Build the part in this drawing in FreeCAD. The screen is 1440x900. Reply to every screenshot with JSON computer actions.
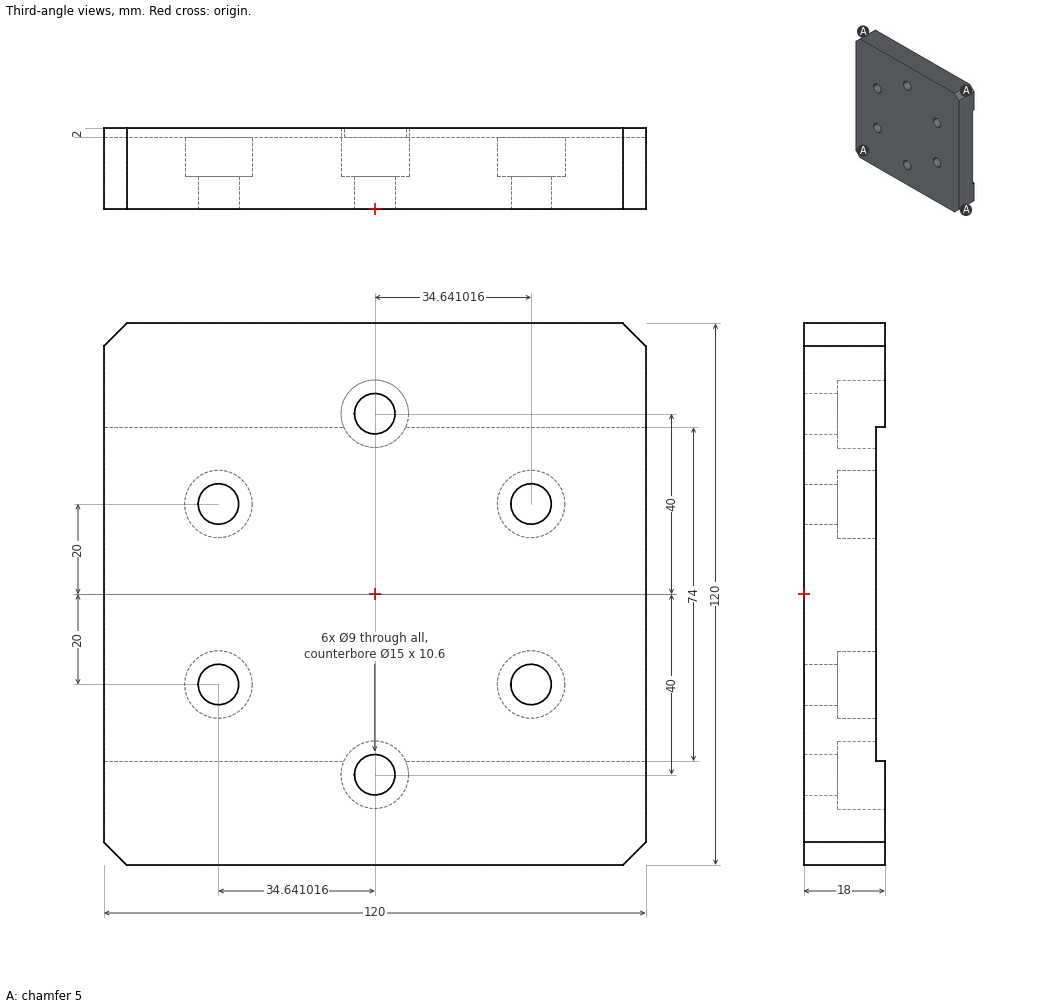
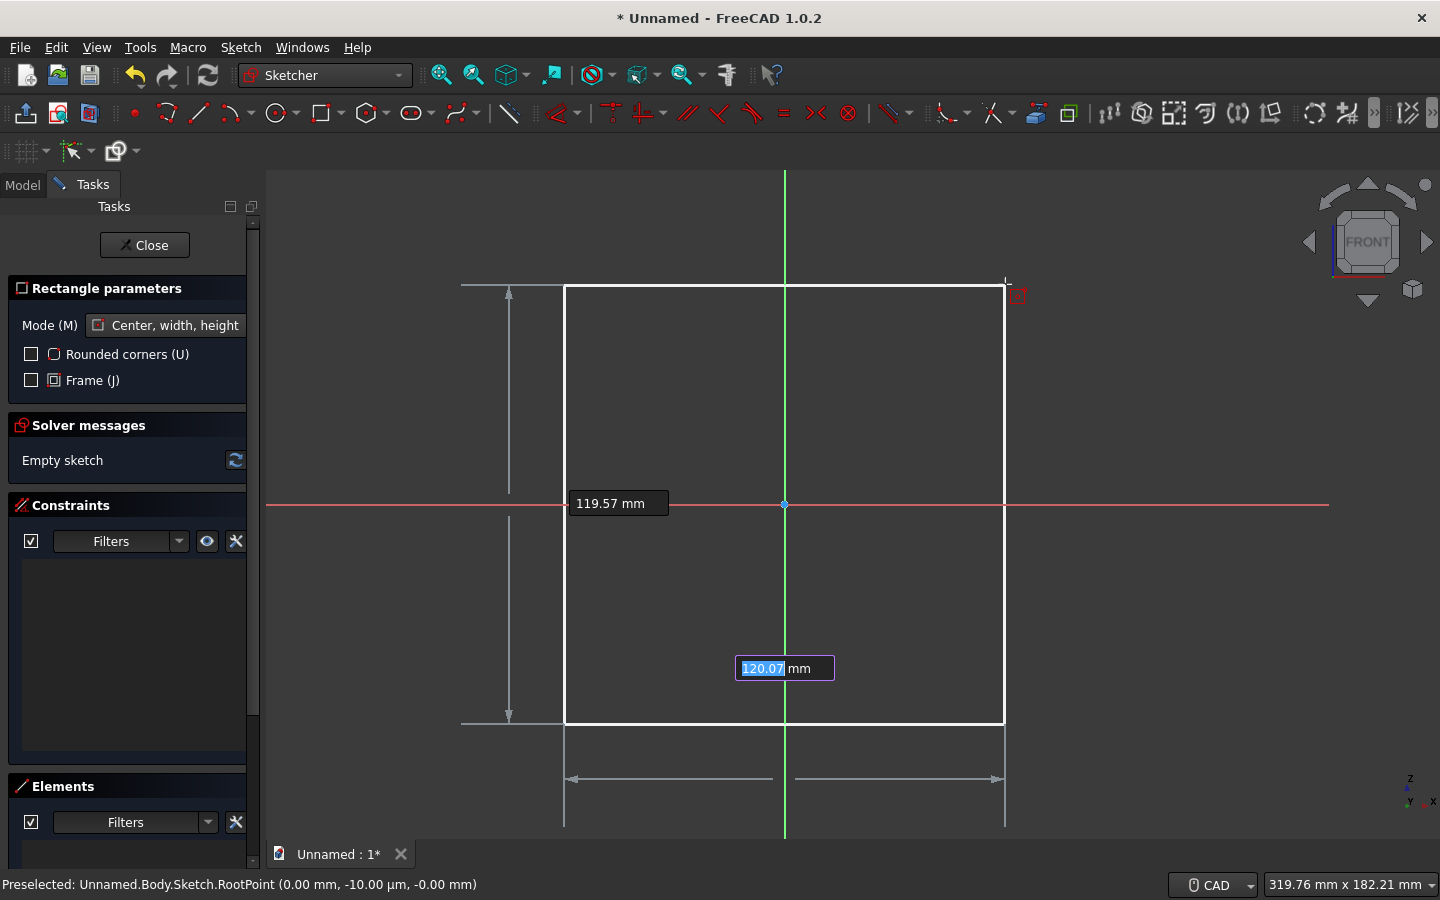
{"action": "type", "text": "120"}
{"action": "key", "text": "Tab"}
{"action": "type", "text": "120"}
{"action": "key", "text": "Return"}
{"action": "key", "text": "Escape"}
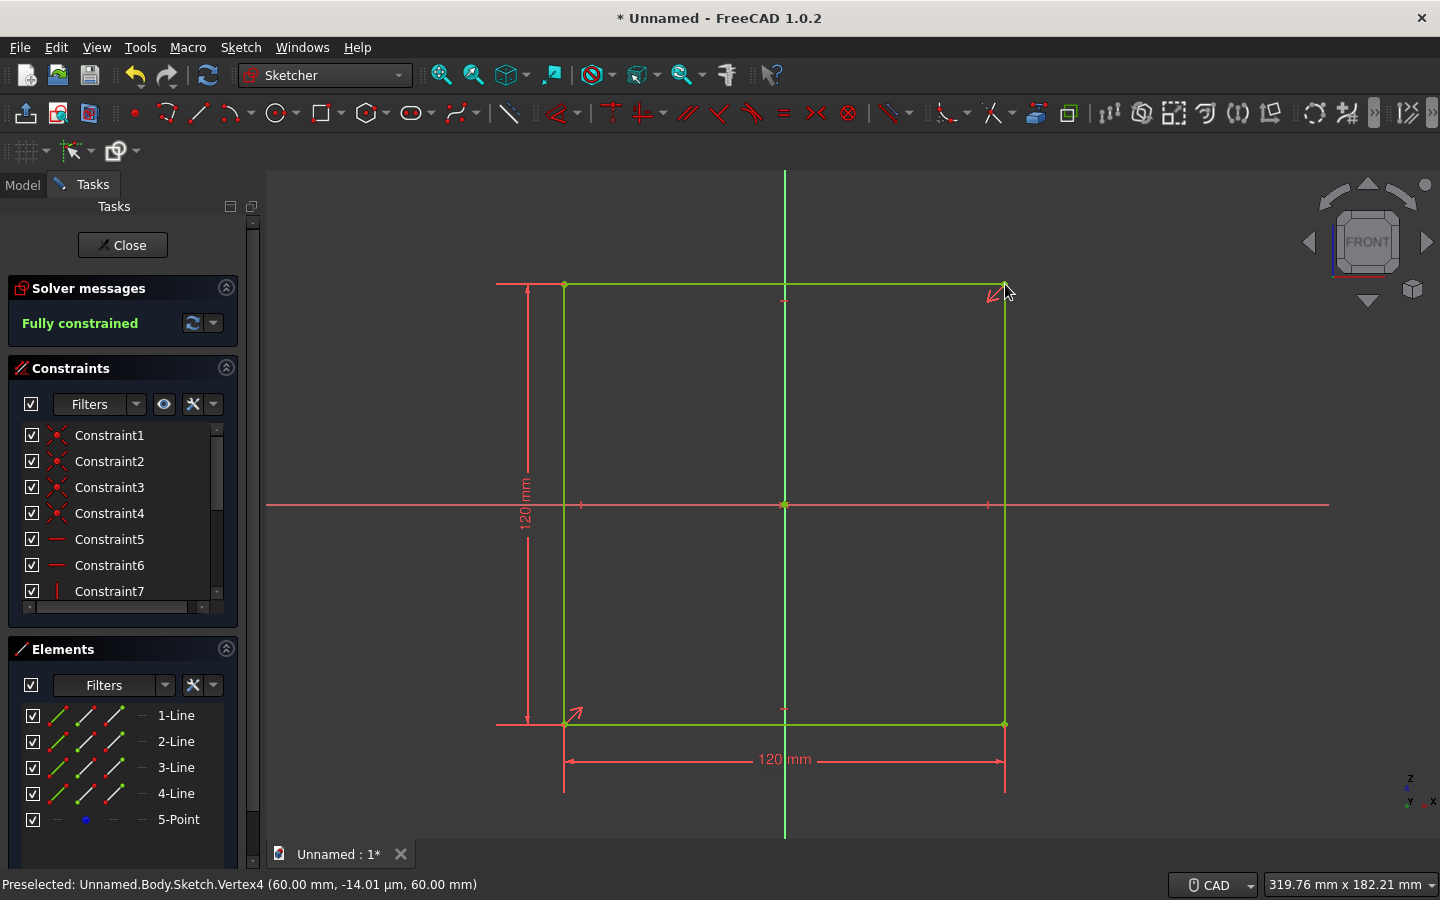
{"action": "left_click", "coordinate": [123, 245]}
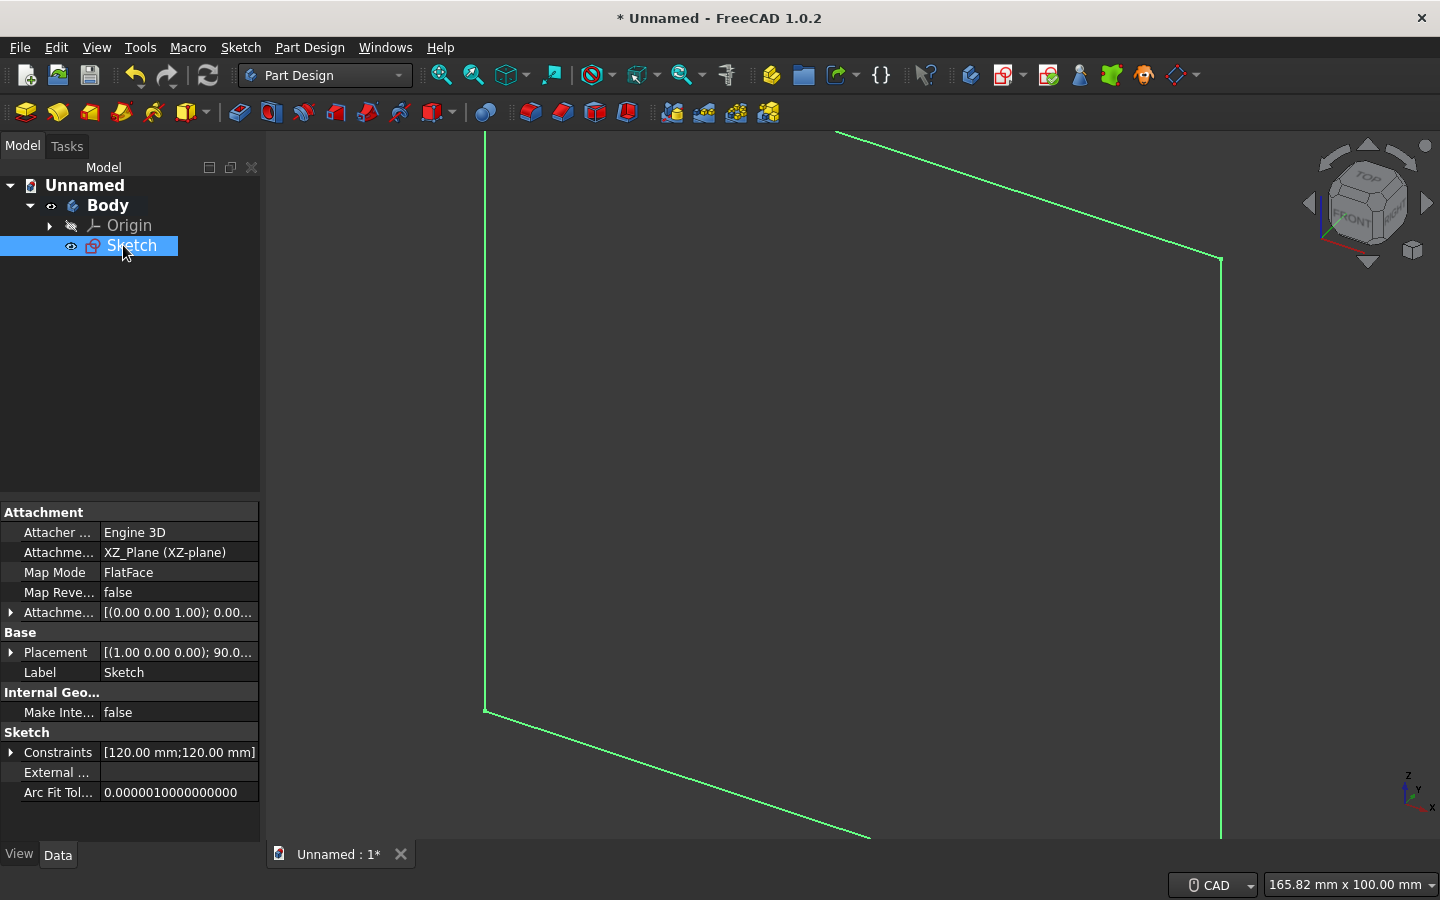
{"action": "left_click", "coordinate": [26, 112]}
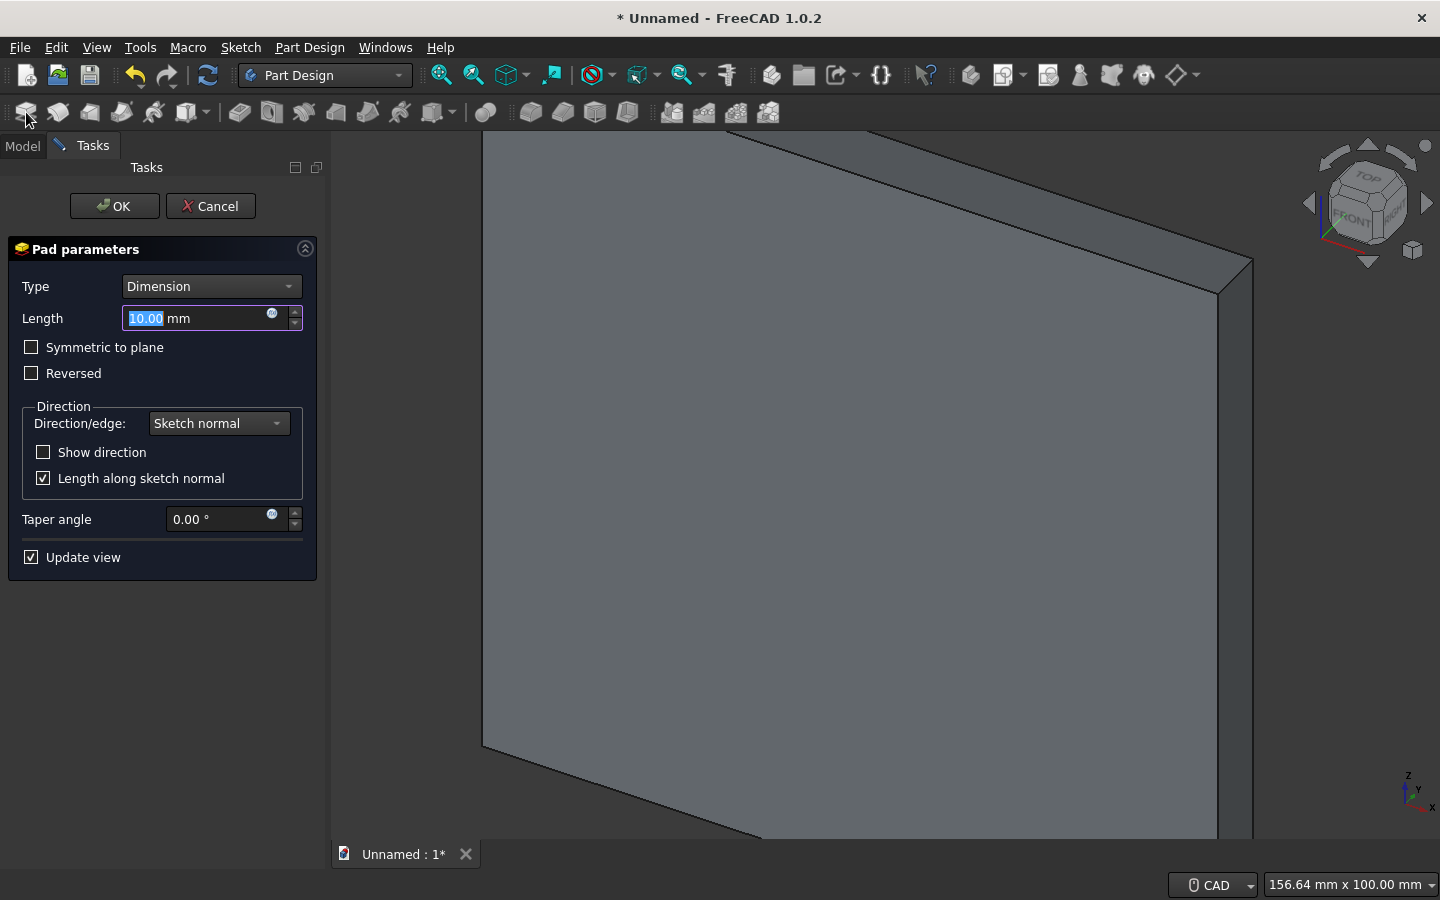
{"action": "type", "text": "18"}
{"action": "key", "text": "Tab"}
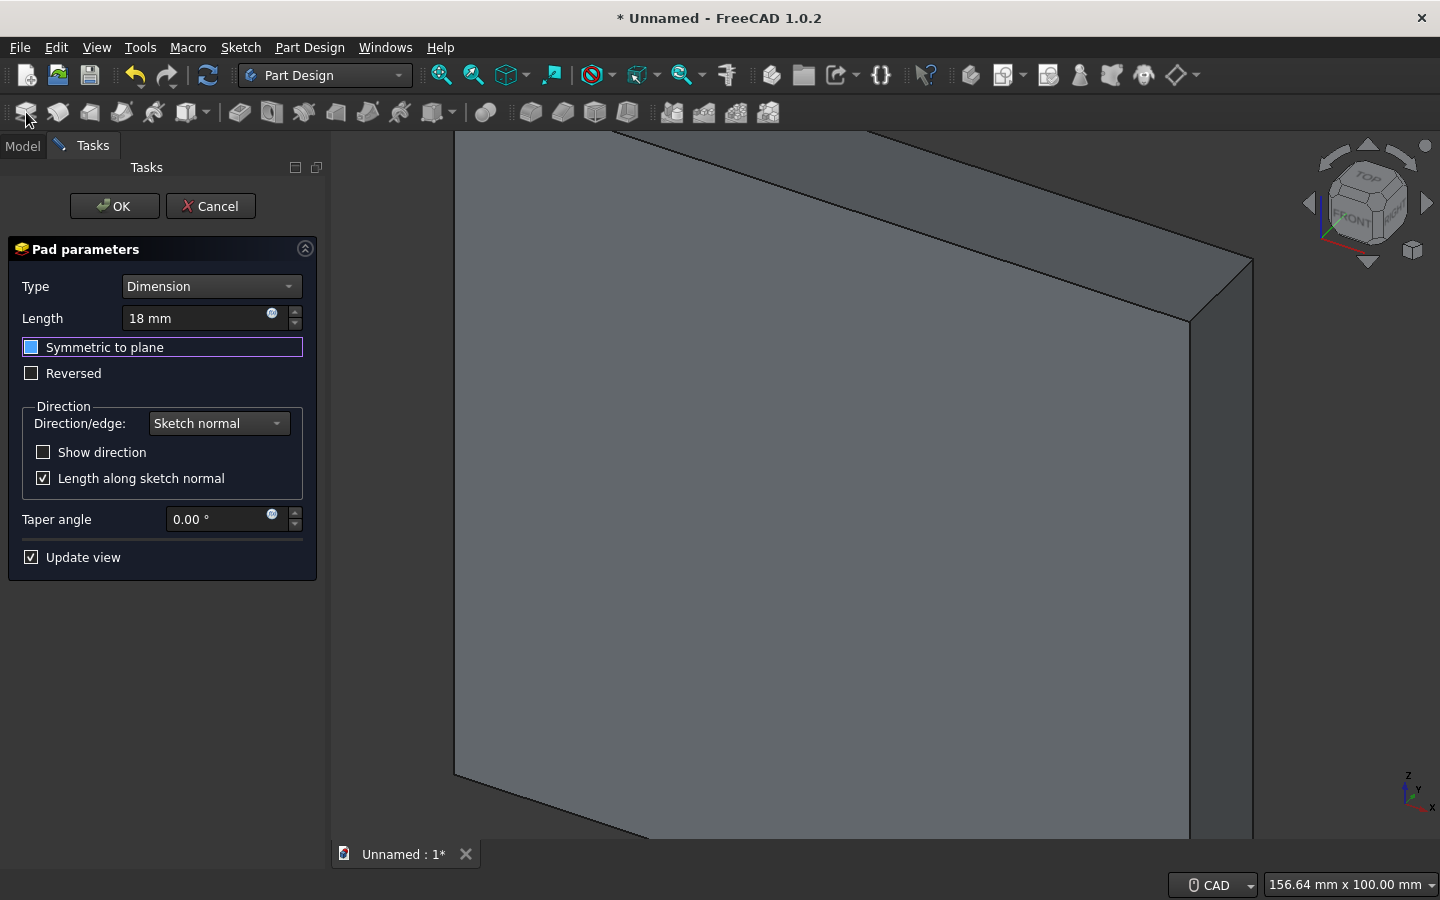
{"action": "left_click", "coordinate": [30, 373]}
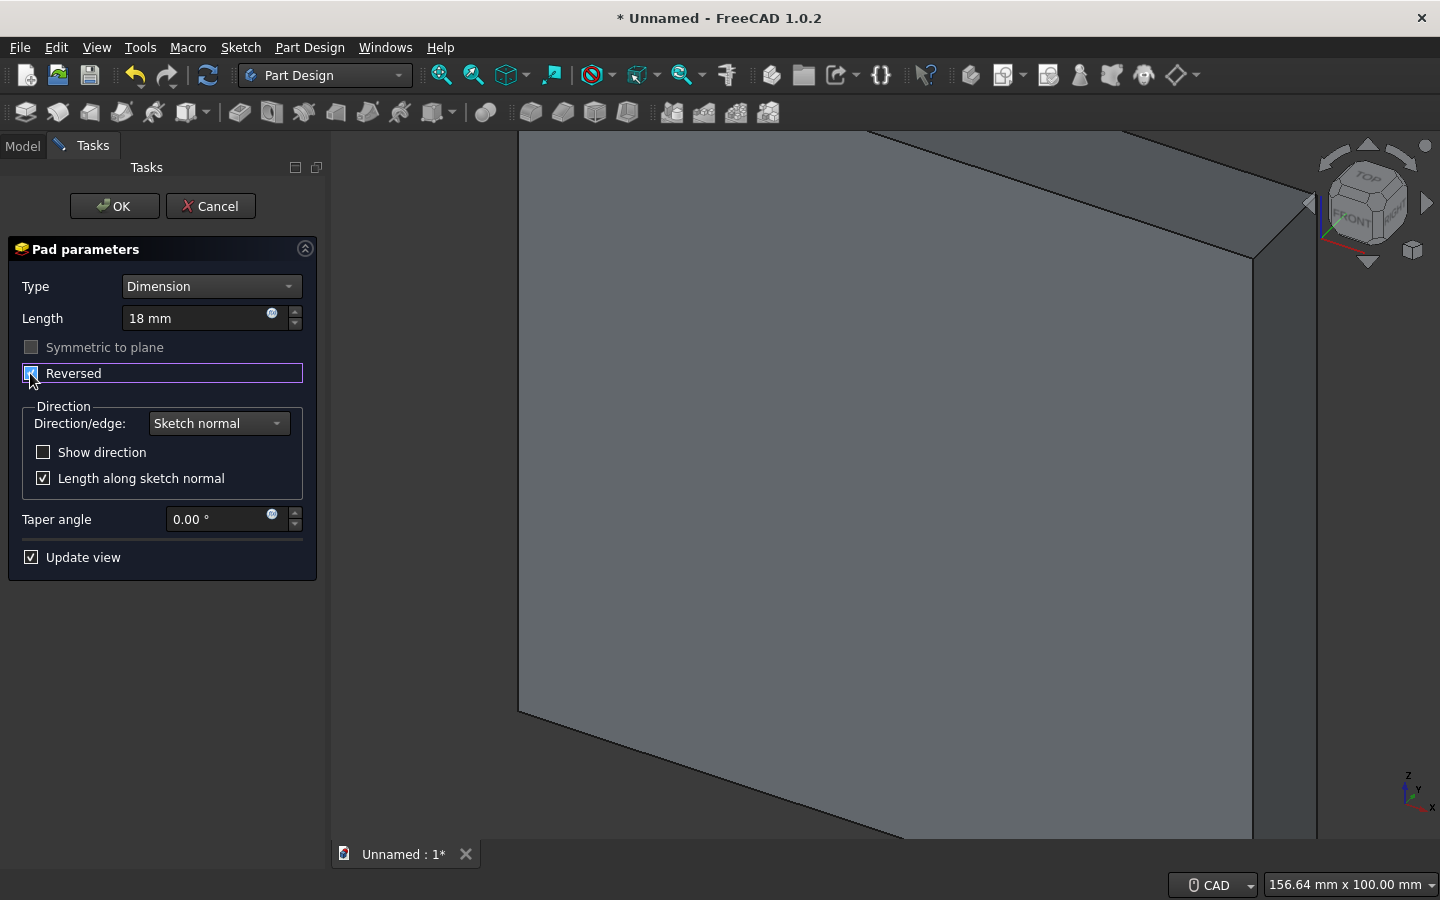
{"action": "left_click", "coordinate": [115, 206]}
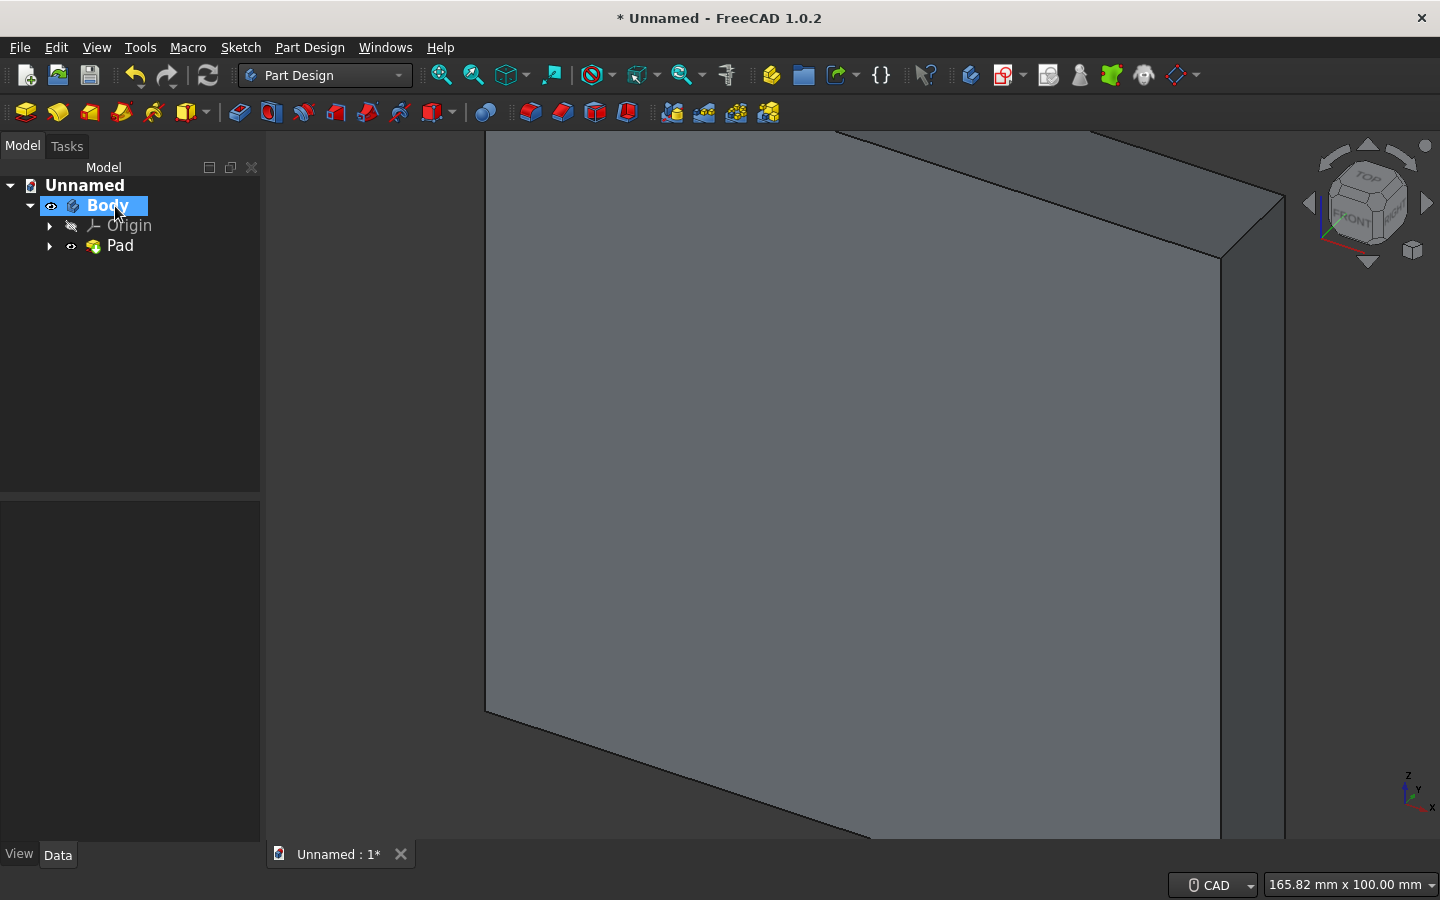
{"action": "left_click", "coordinate": [442, 76]}